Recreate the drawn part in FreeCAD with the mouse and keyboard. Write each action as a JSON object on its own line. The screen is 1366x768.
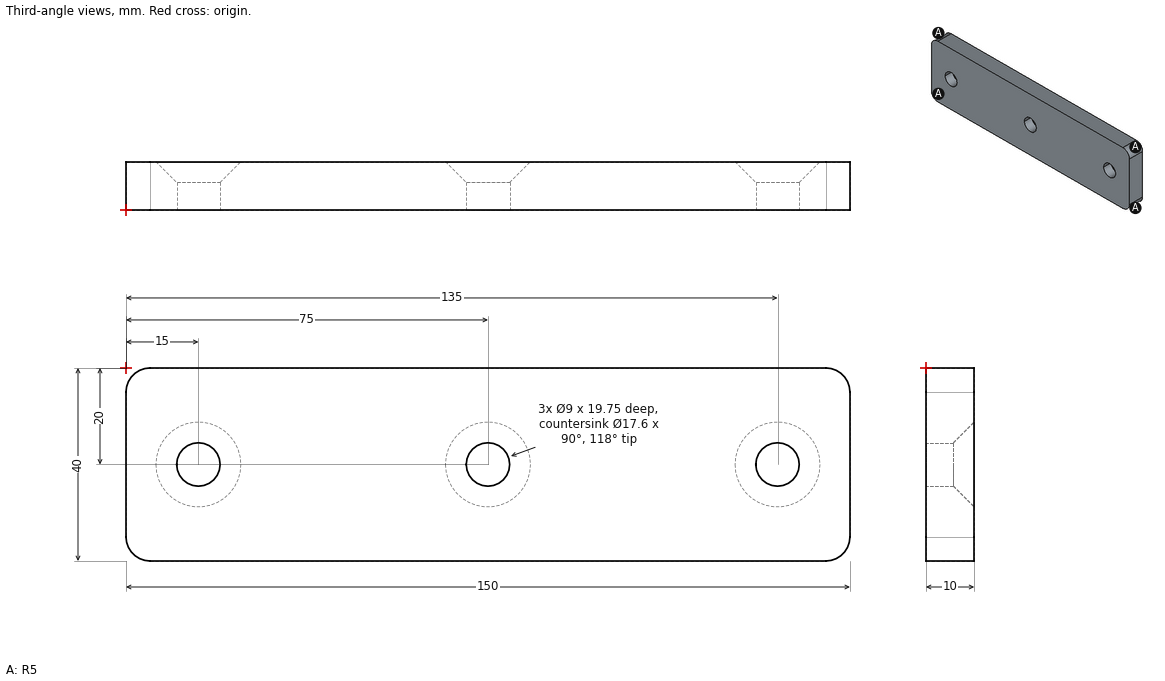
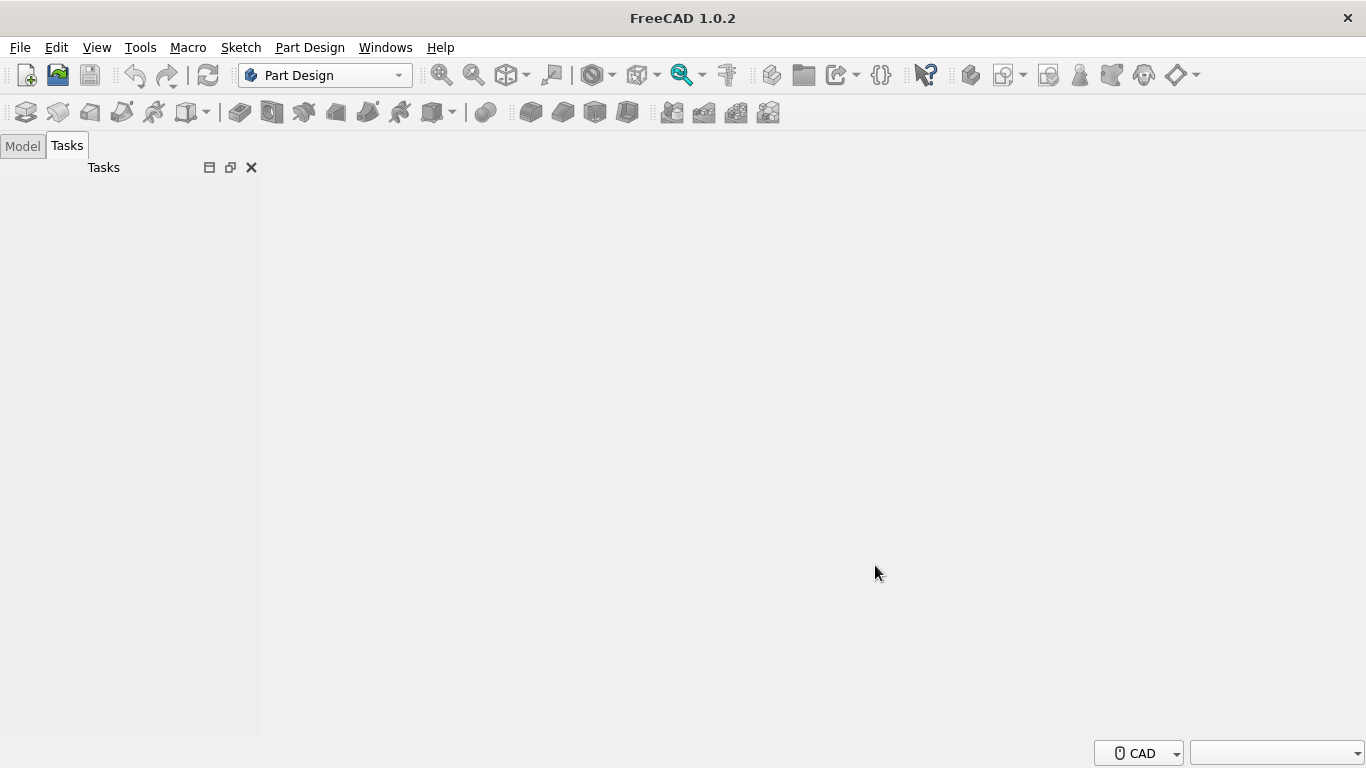
{"action": "left_click", "coordinate": [26, 76]}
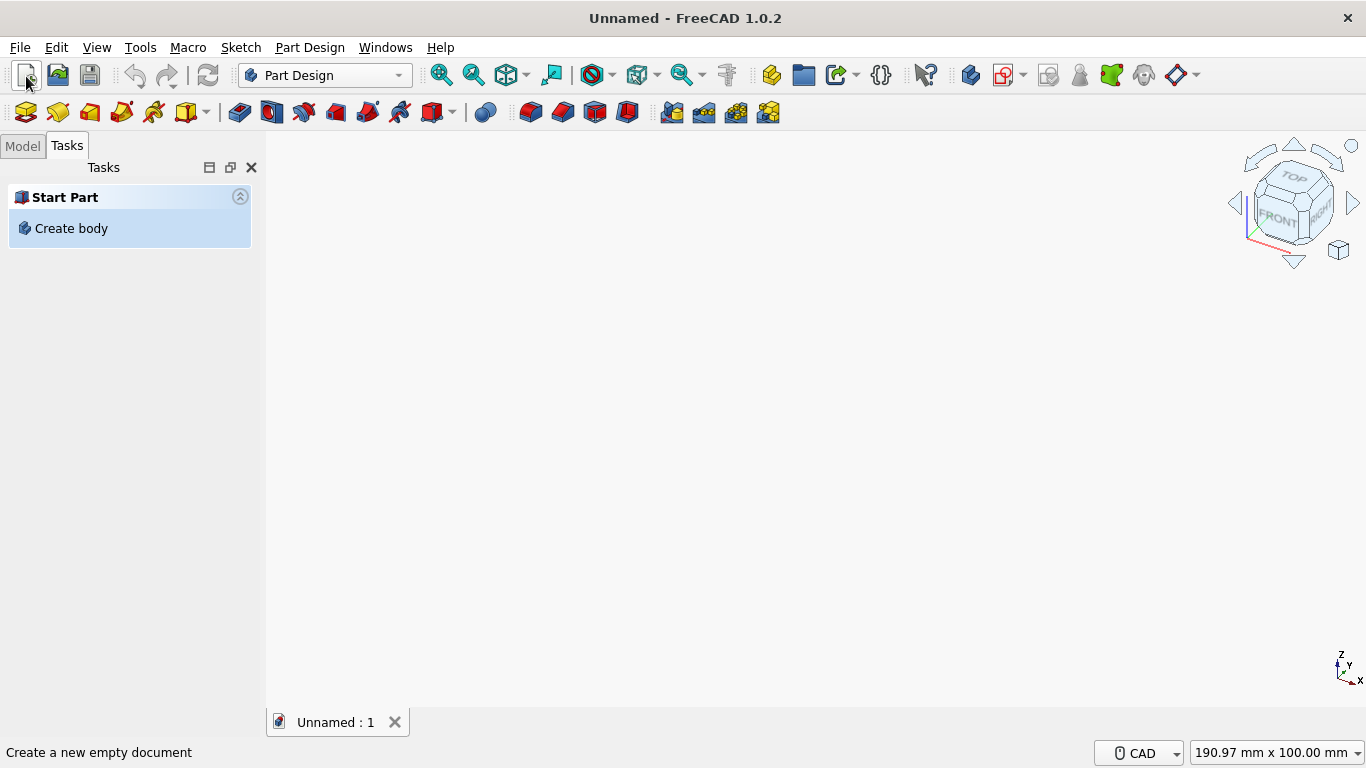
{"action": "left_click", "coordinate": [1004, 76]}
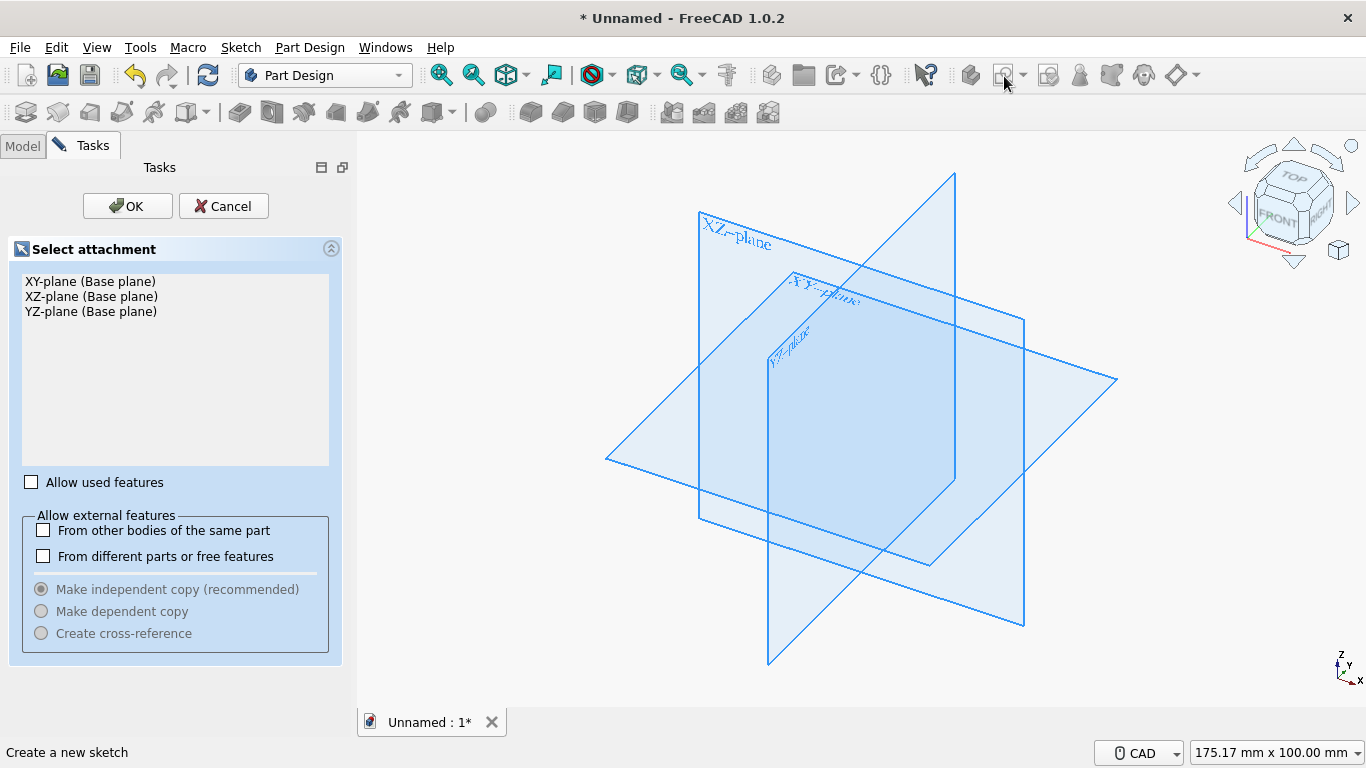
{"action": "left_click", "coordinate": [82, 296]}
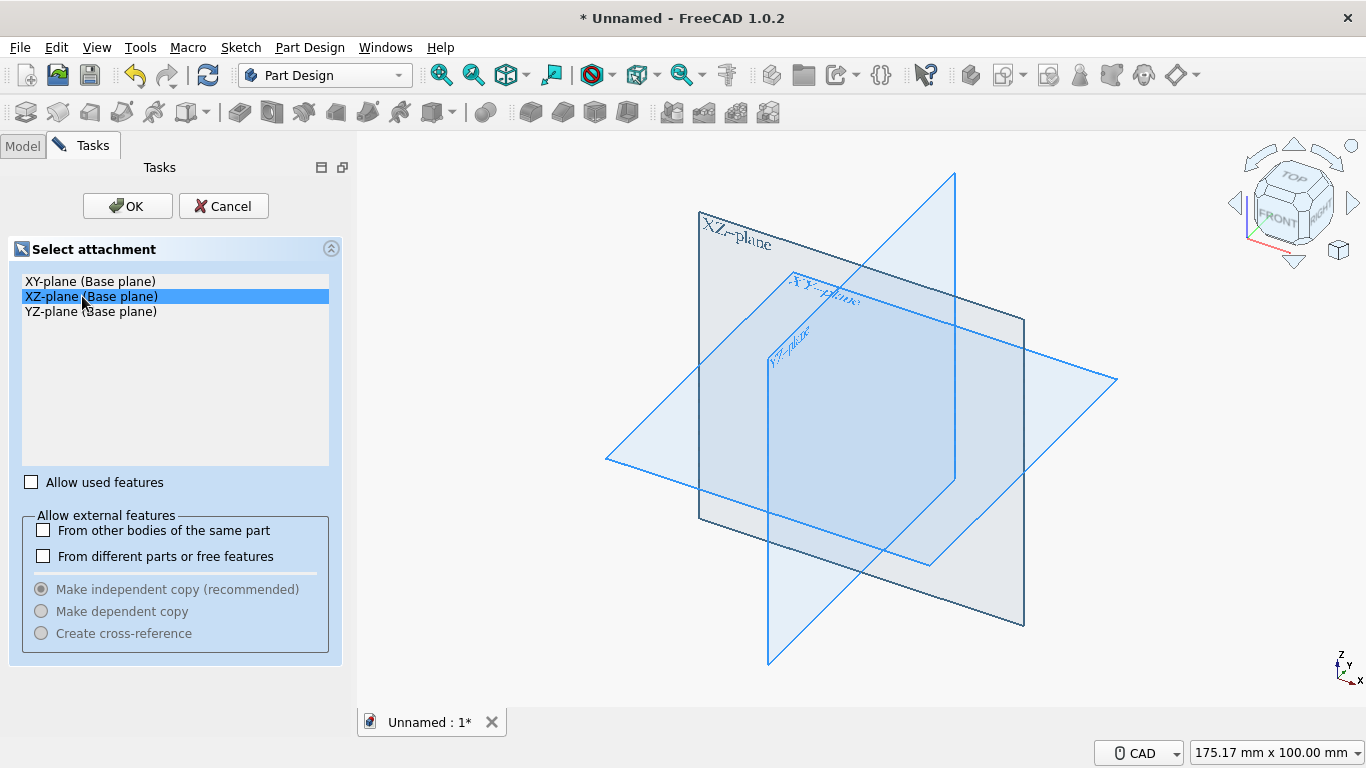
{"action": "left_click", "coordinate": [128, 206]}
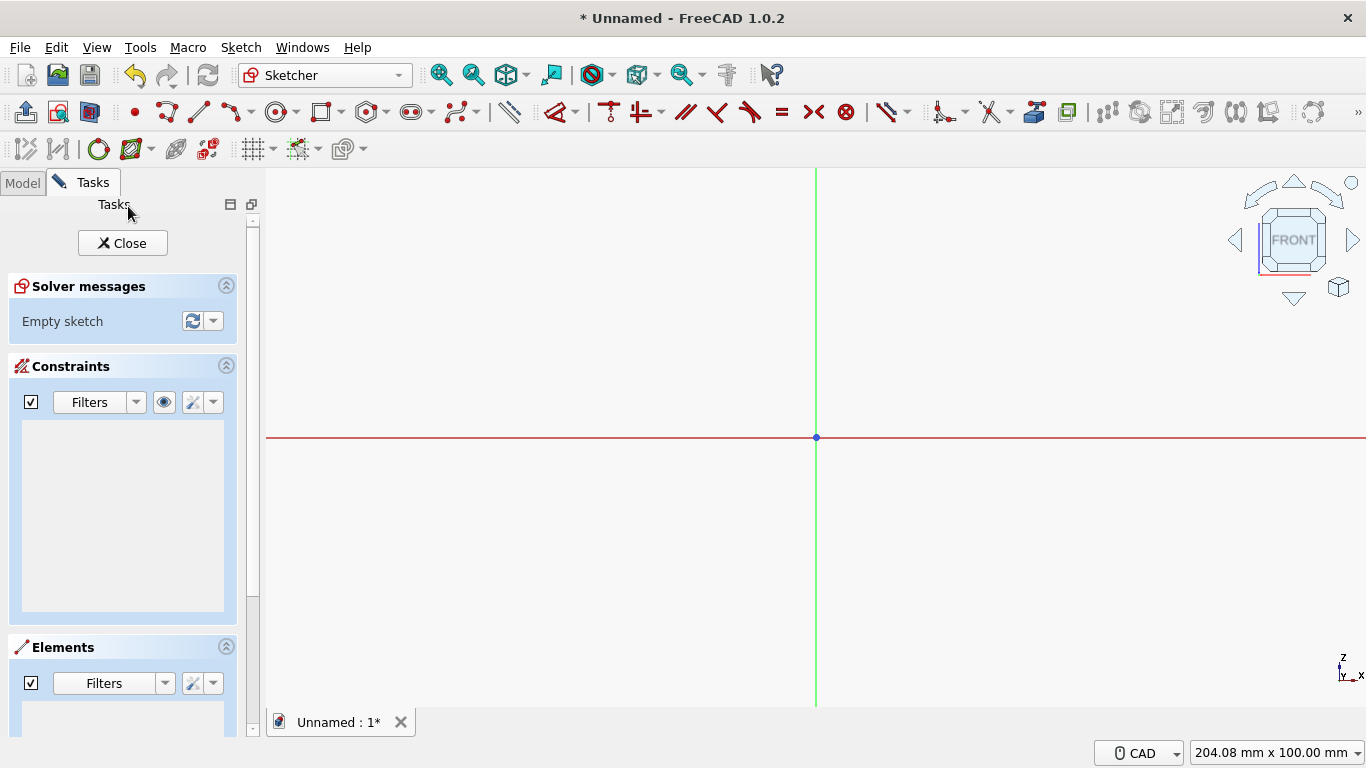
{"action": "scroll", "coordinate": [294, 306], "scroll_direction": "down", "scroll_amount": 3}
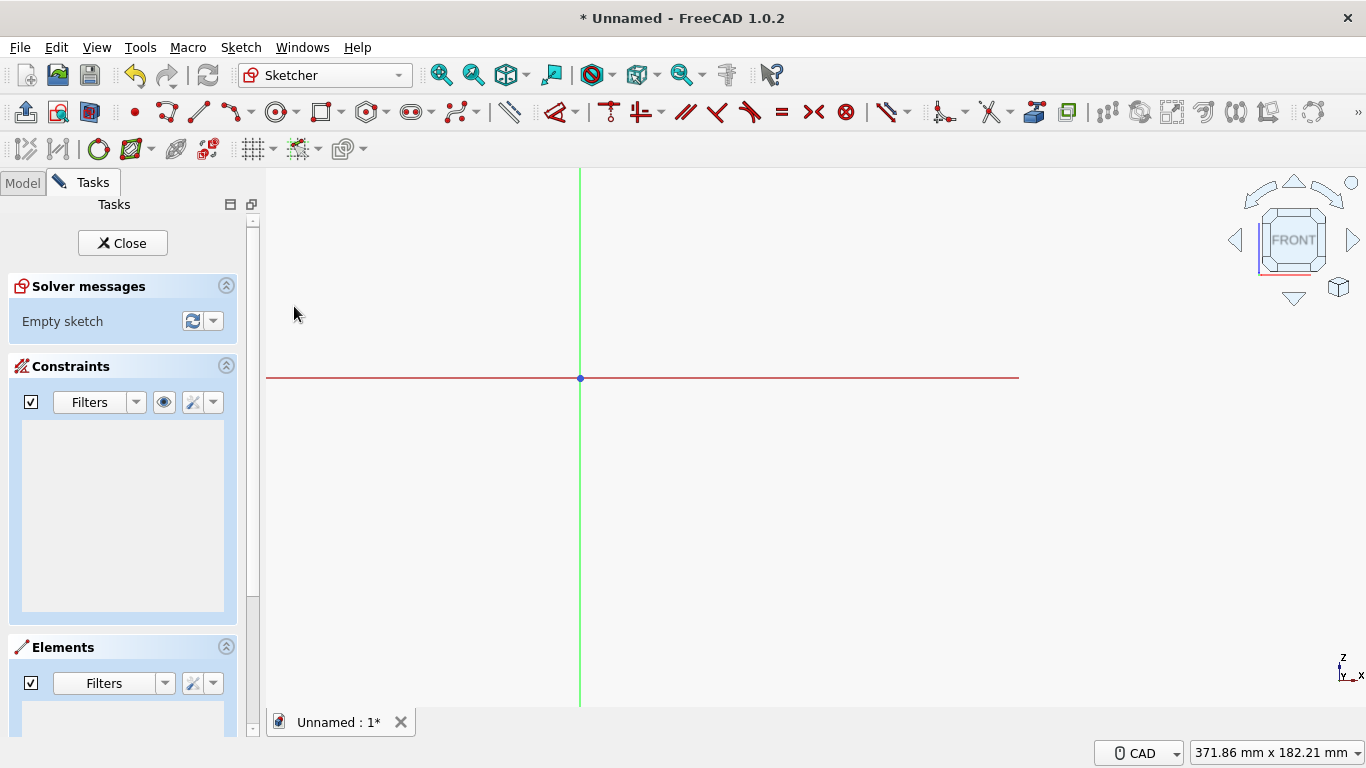
{"action": "scroll", "coordinate": [914, 437], "scroll_direction": "up", "scroll_amount": 2}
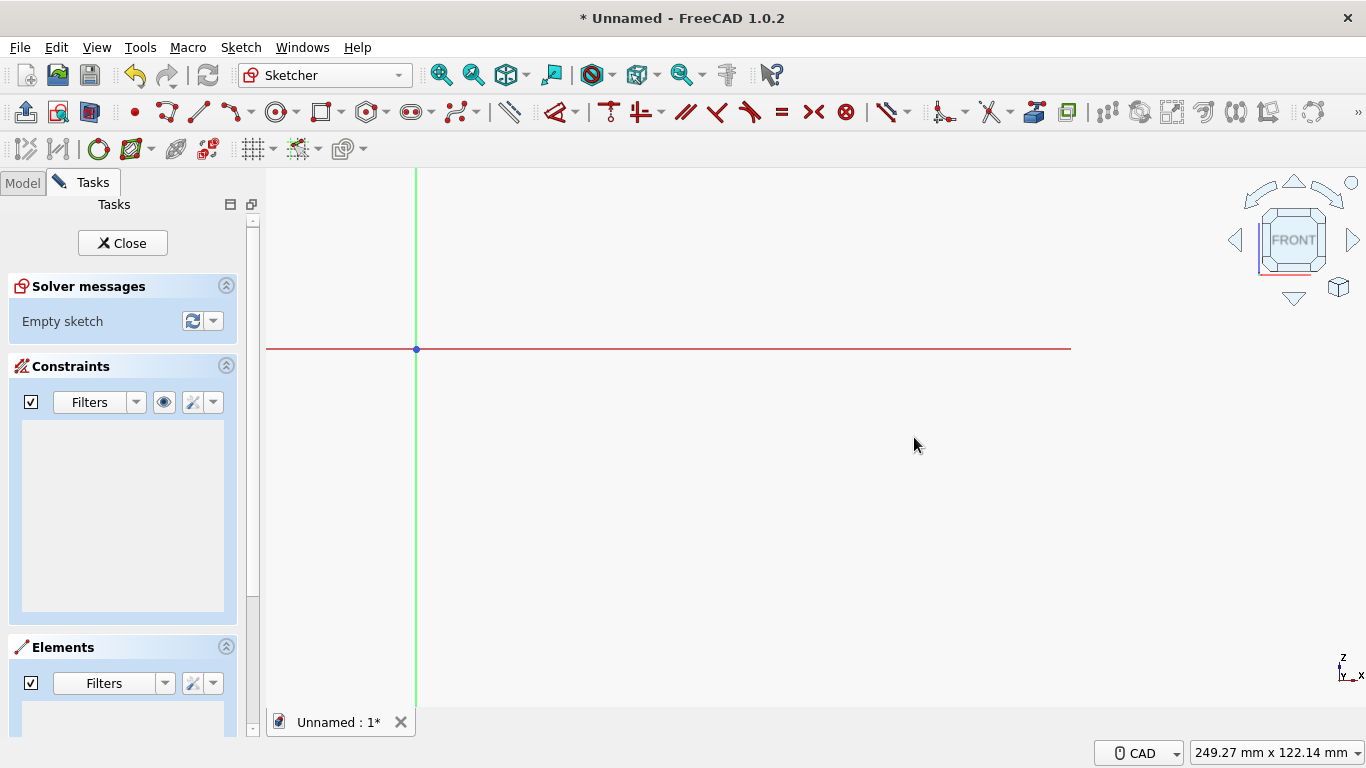
{"action": "left_click", "coordinate": [322, 112]}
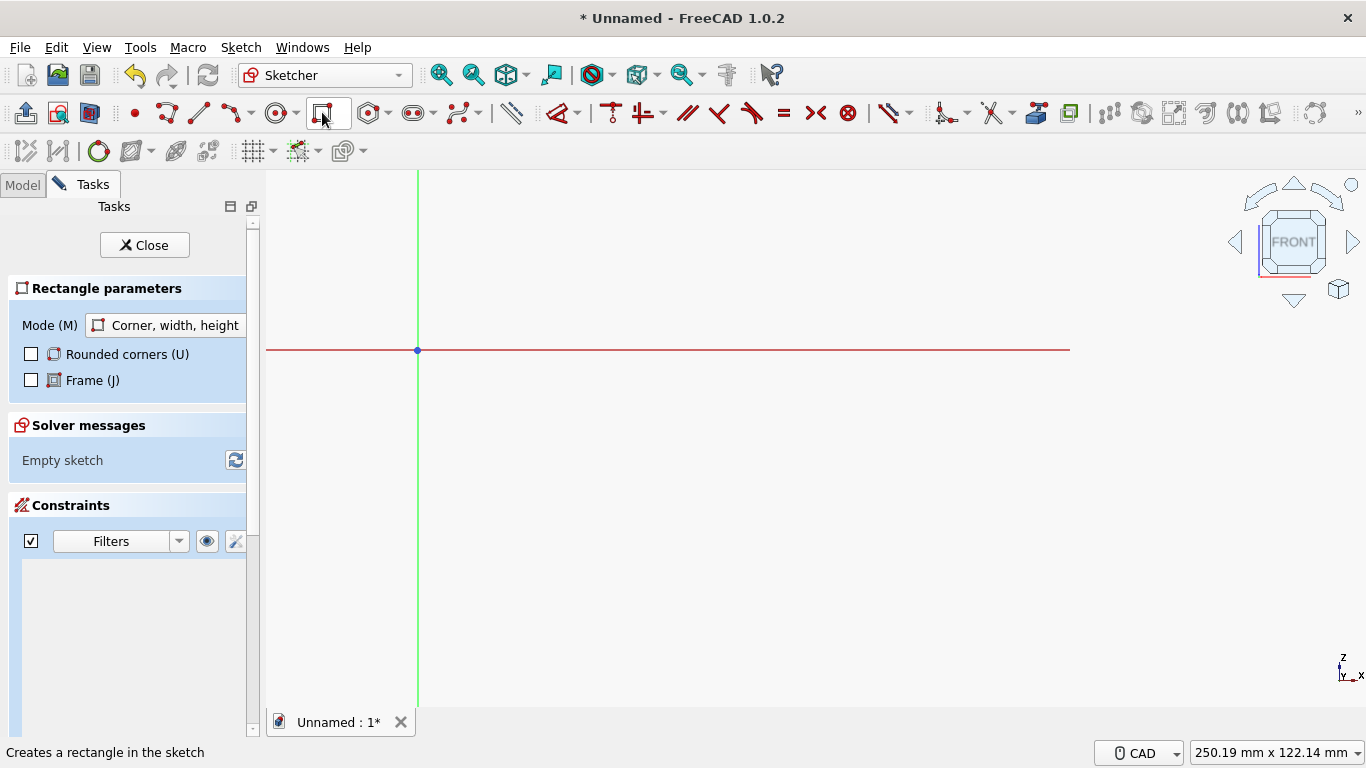
{"action": "left_click", "coordinate": [418, 350]}
{"action": "left_click", "coordinate": [1077, 526]}
{"action": "key", "text": "Escape"}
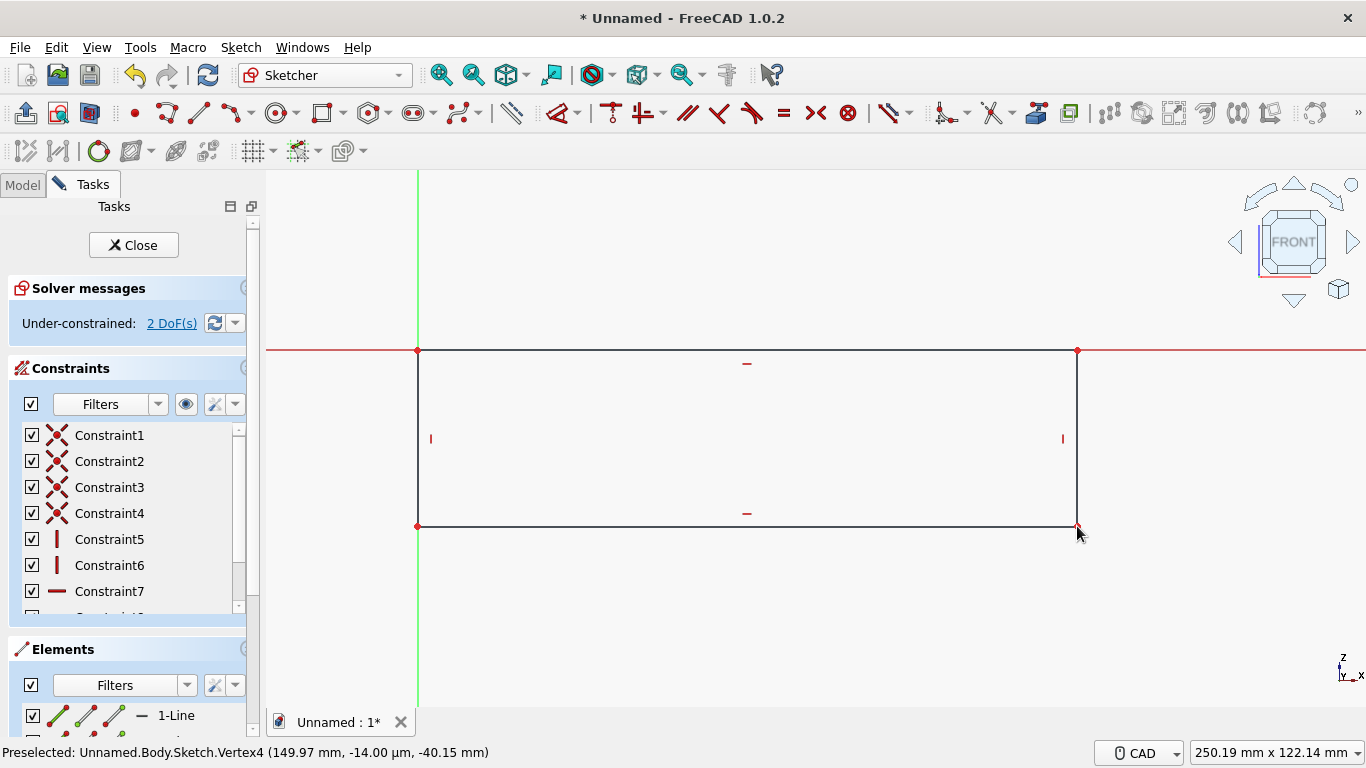
{"action": "left_click", "coordinate": [558, 114]}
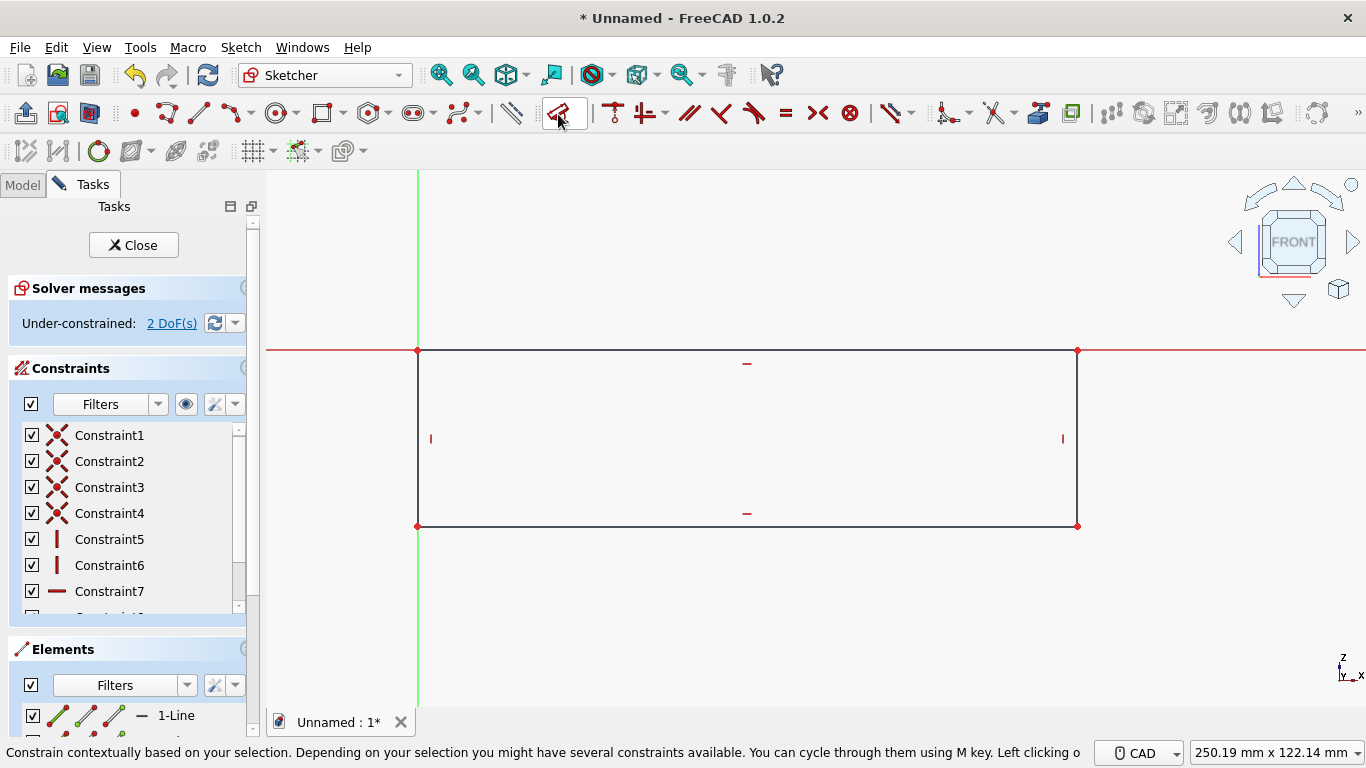
{"action": "left_click", "coordinate": [418, 403]}
{"action": "left_click", "coordinate": [384, 439]}